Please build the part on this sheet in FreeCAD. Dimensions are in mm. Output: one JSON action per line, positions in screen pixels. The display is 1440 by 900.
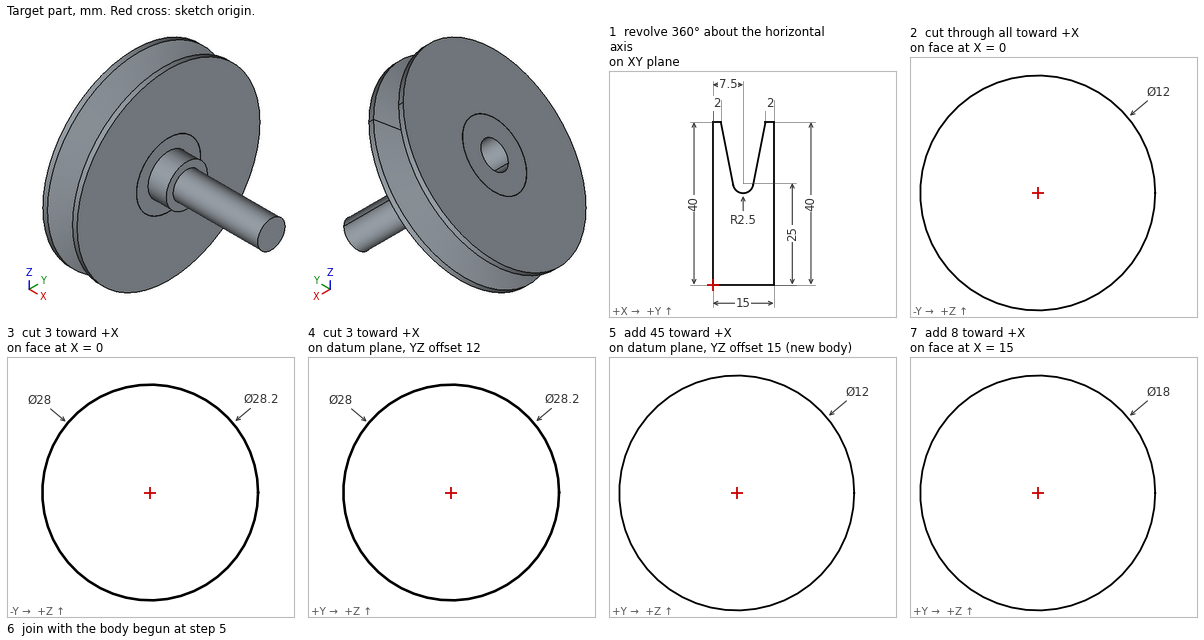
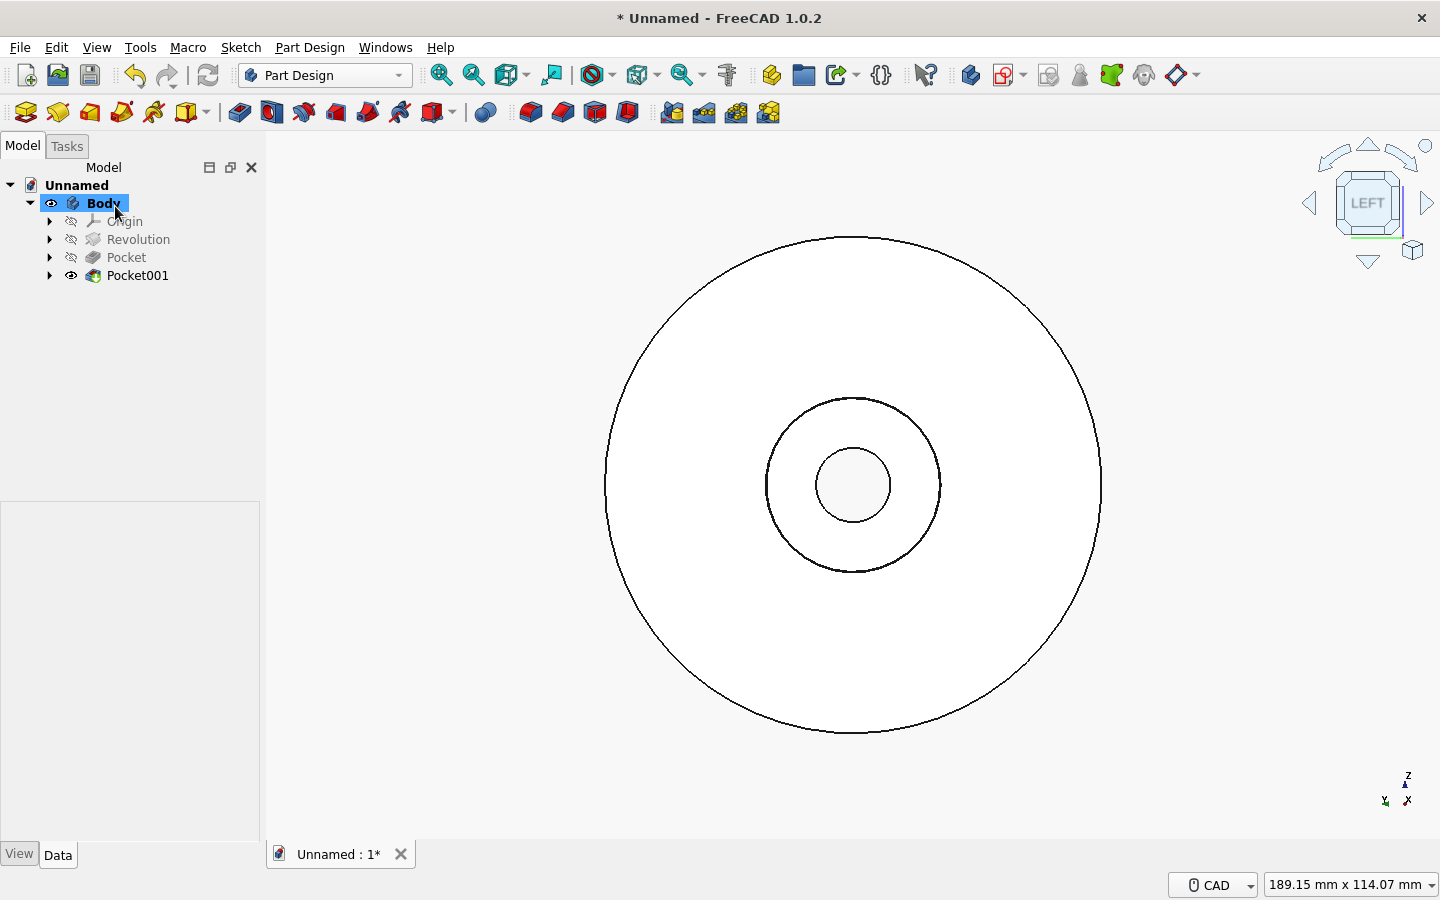
{"action": "left_click", "coordinate": [50, 221]}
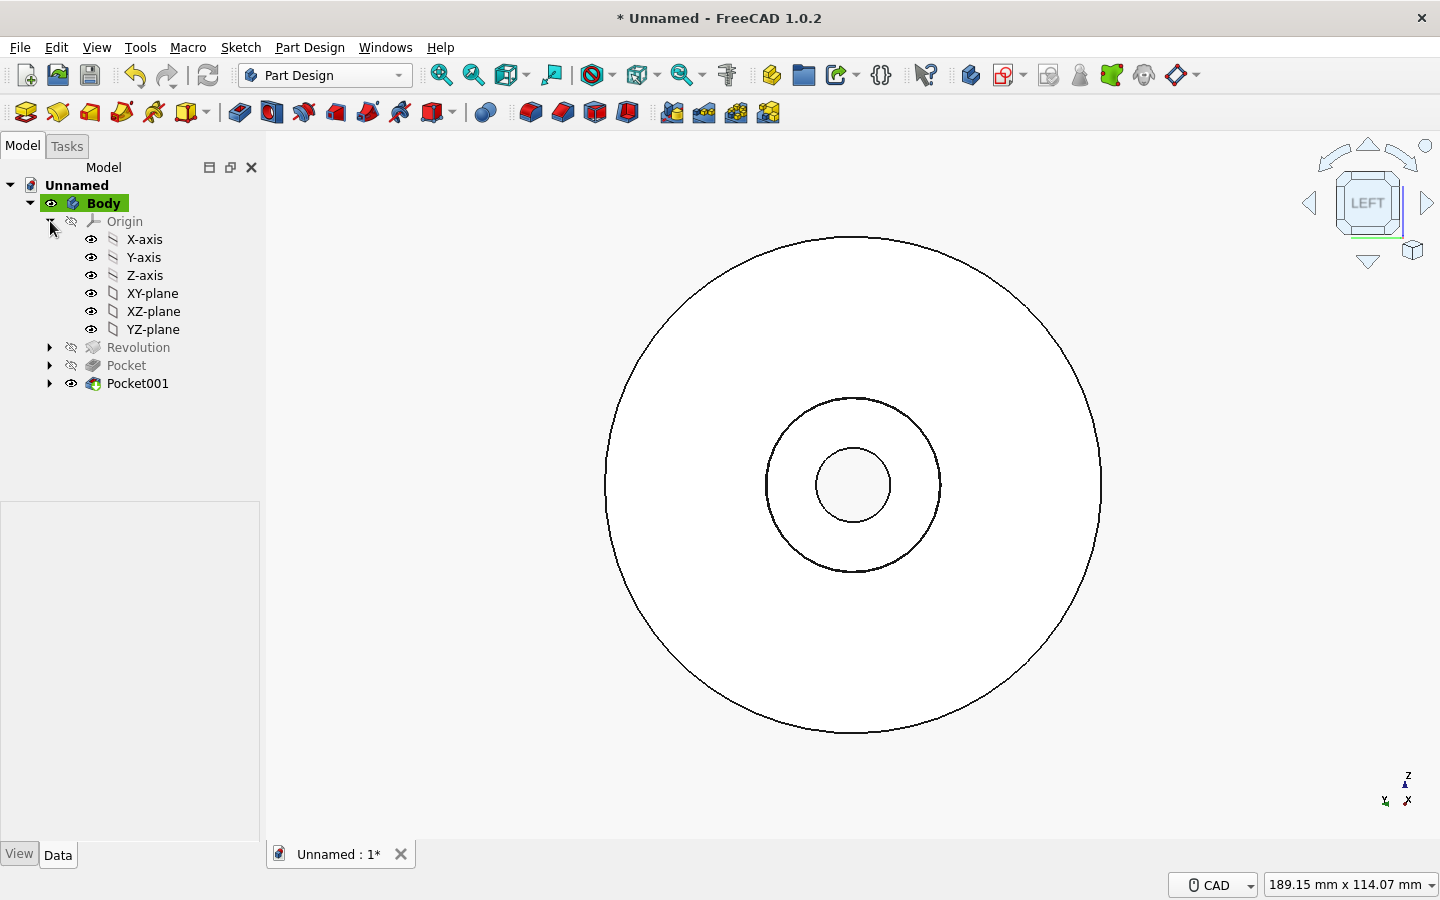
{"action": "left_click", "coordinate": [136, 329]}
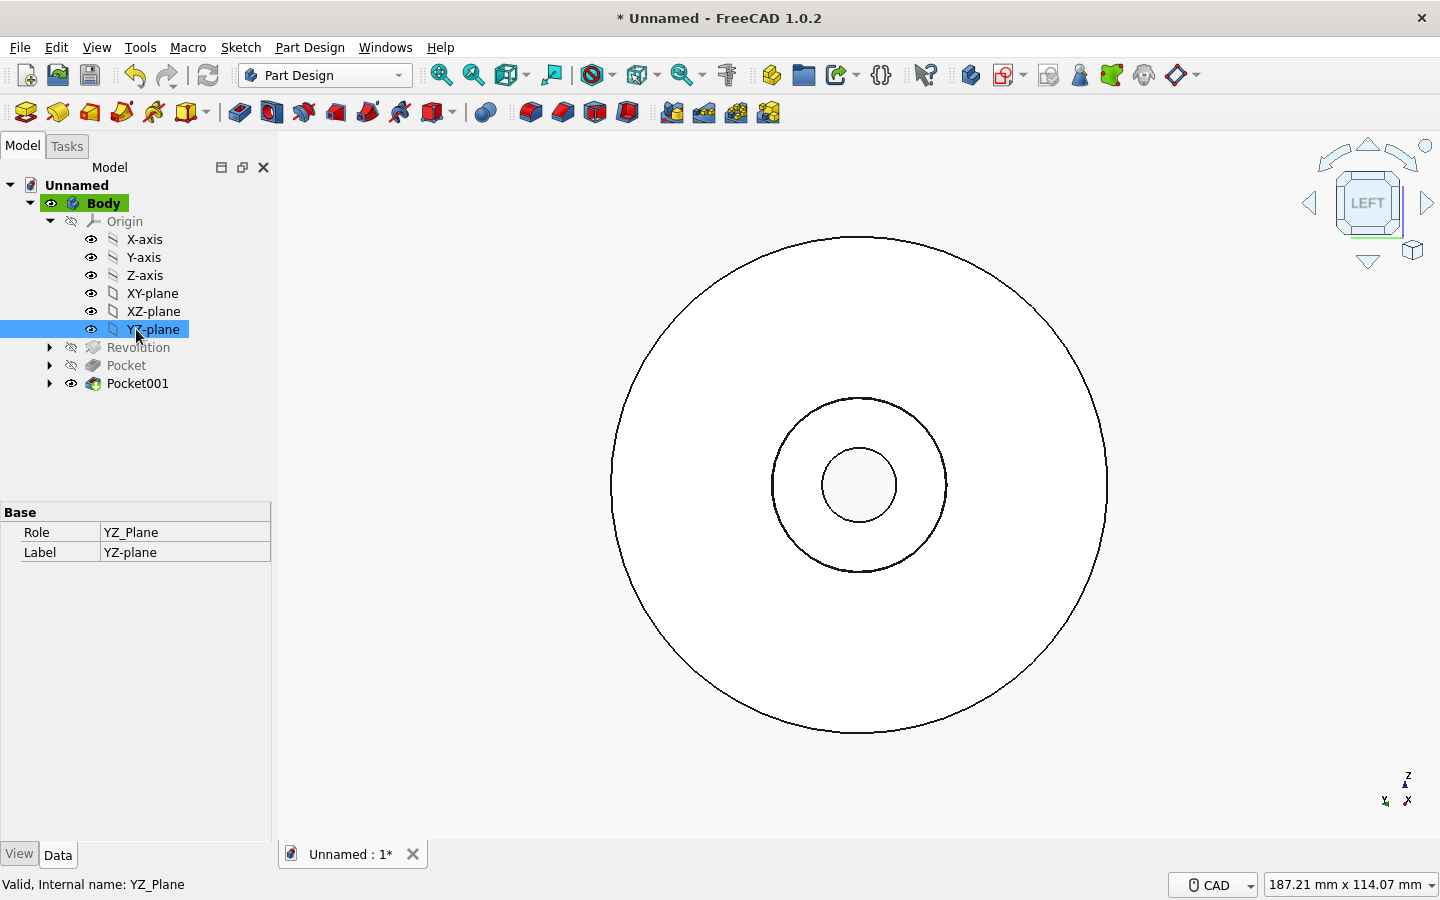
{"action": "left_click", "coordinate": [1176, 76]}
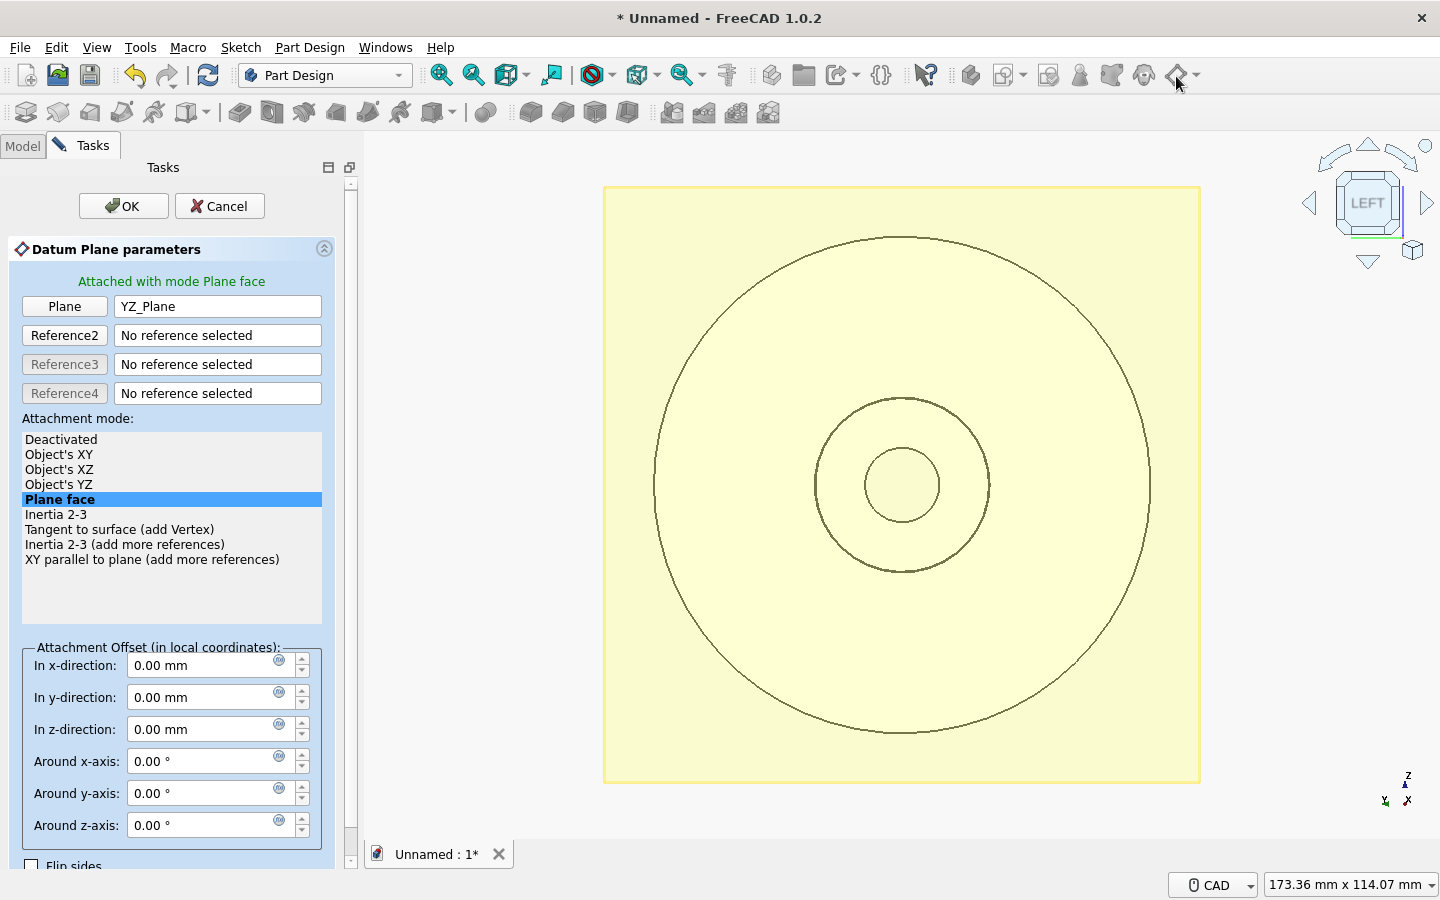
{"action": "triple_click", "coordinate": [210, 729]}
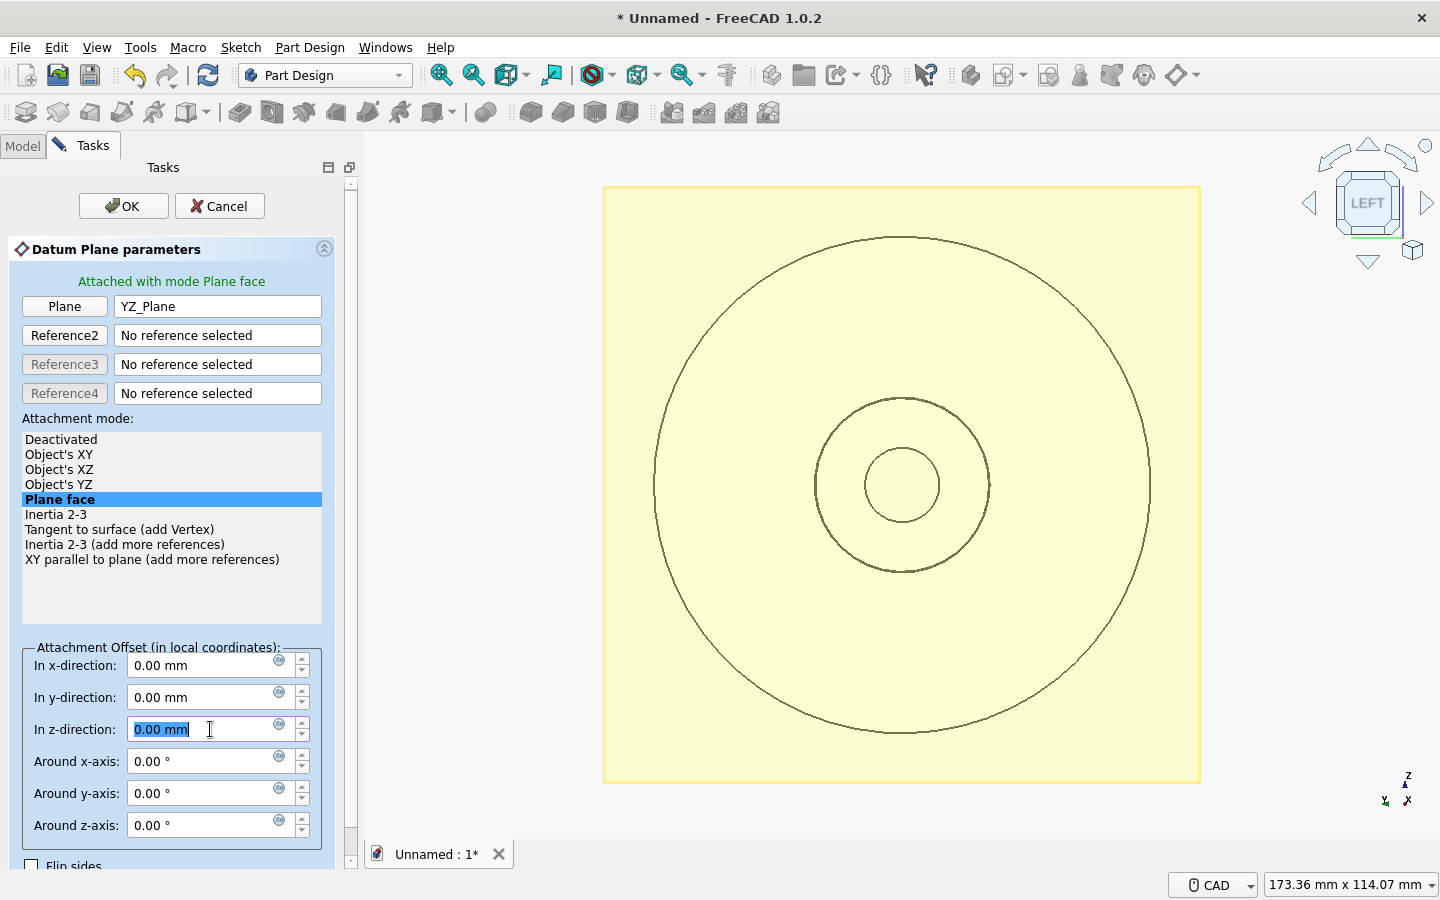
{"action": "type", "text": "12"}
{"action": "key", "text": "Tab"}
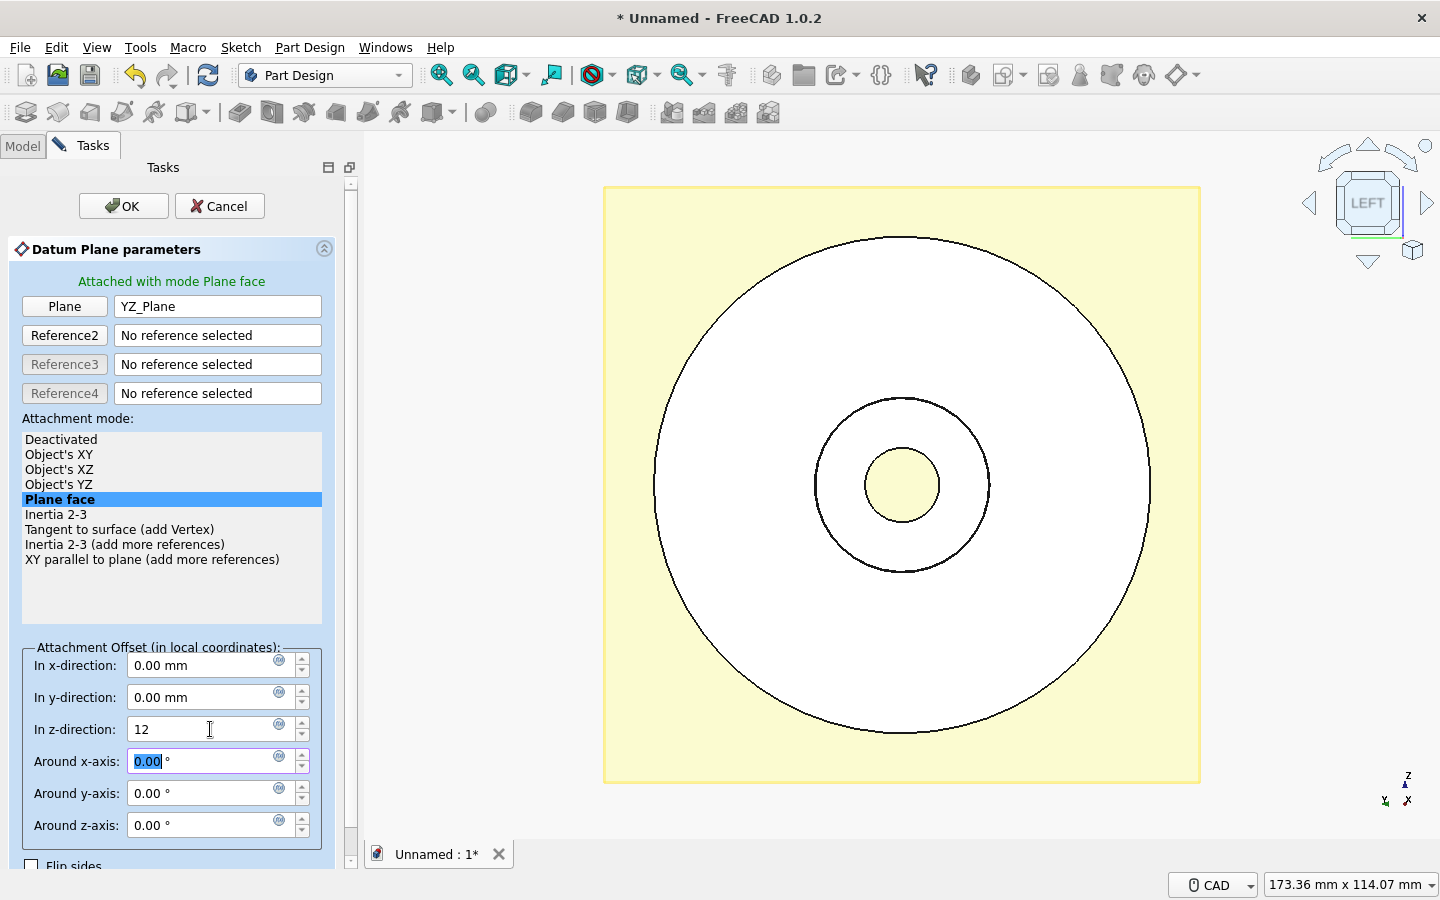
{"action": "left_click", "coordinate": [124, 206]}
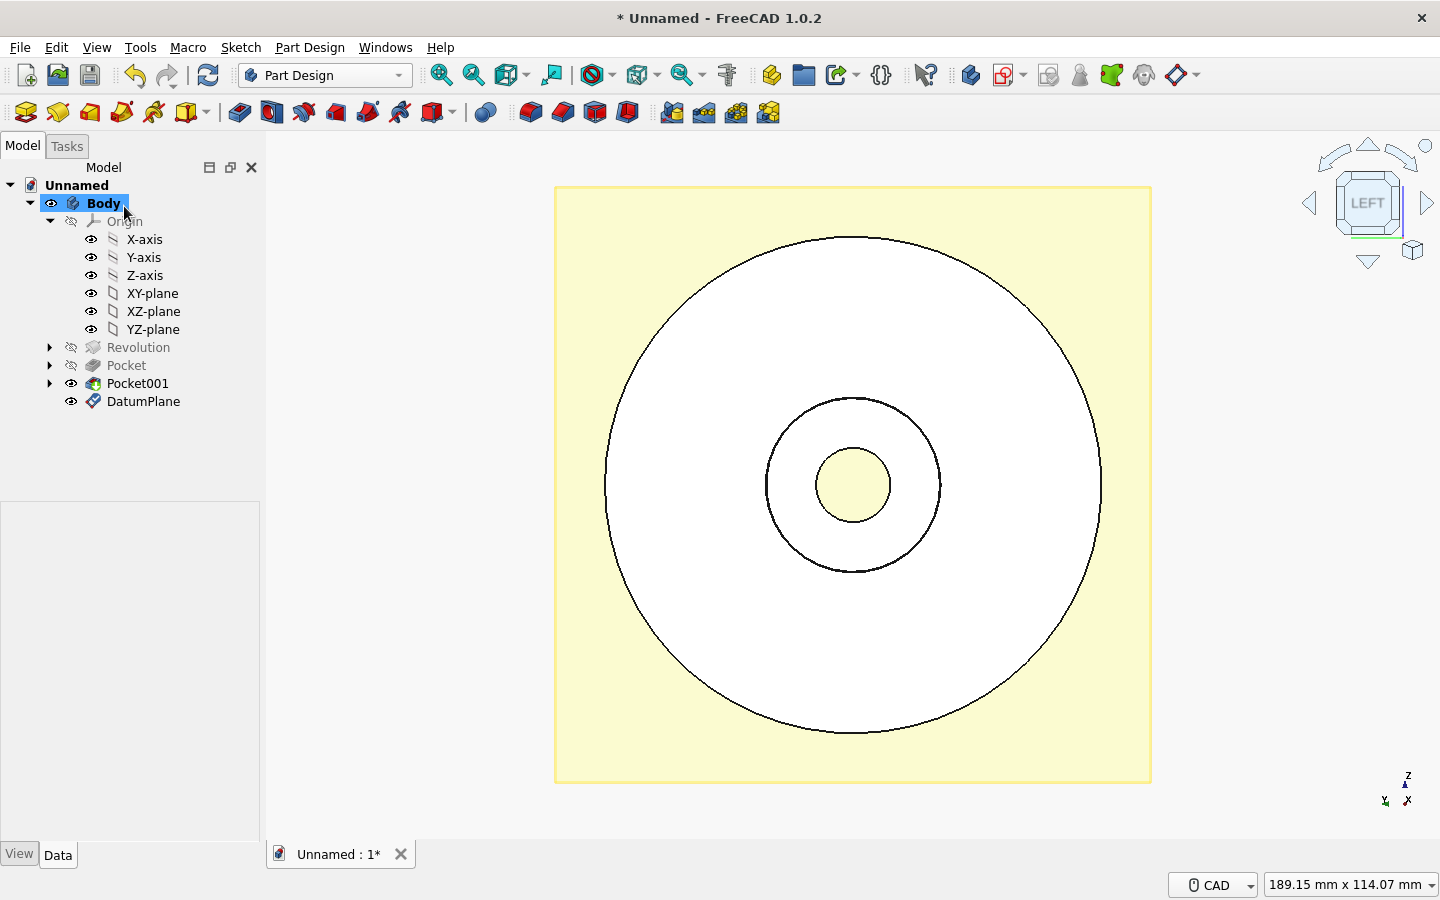
{"action": "left_click", "coordinate": [116, 401]}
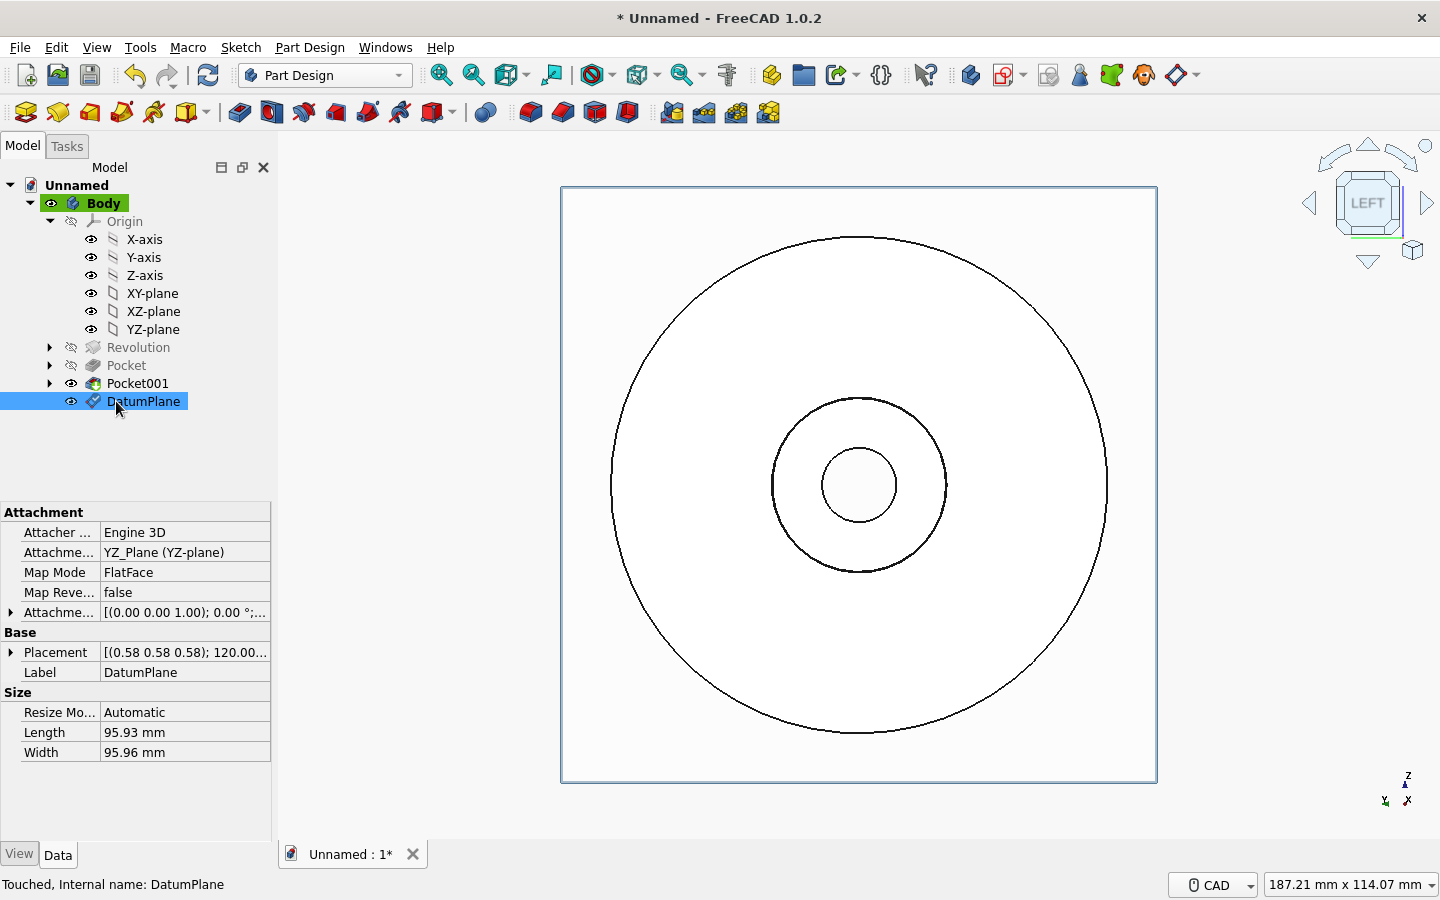
{"action": "left_click", "coordinate": [1004, 76]}